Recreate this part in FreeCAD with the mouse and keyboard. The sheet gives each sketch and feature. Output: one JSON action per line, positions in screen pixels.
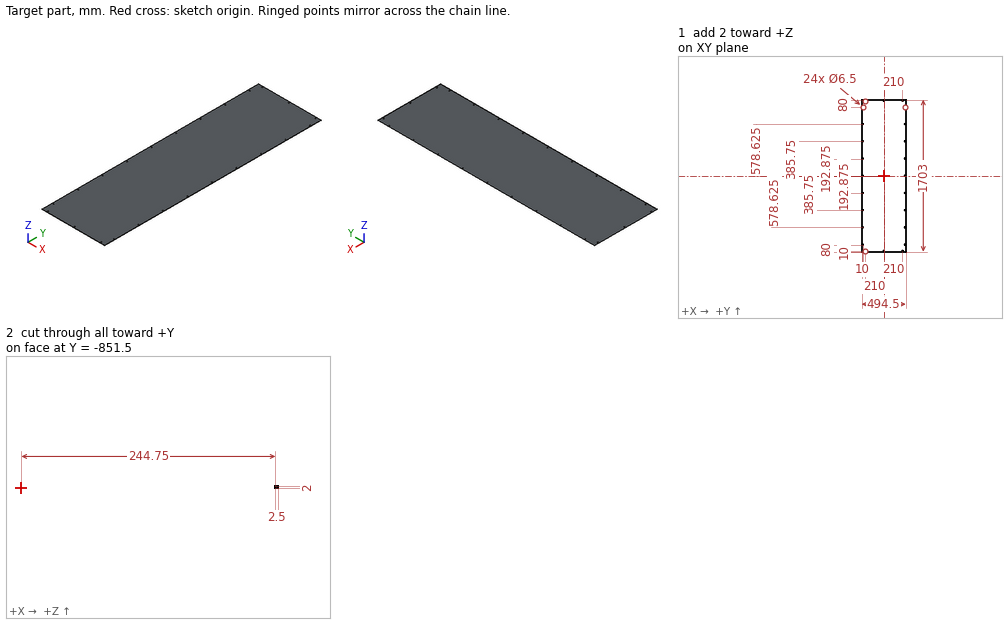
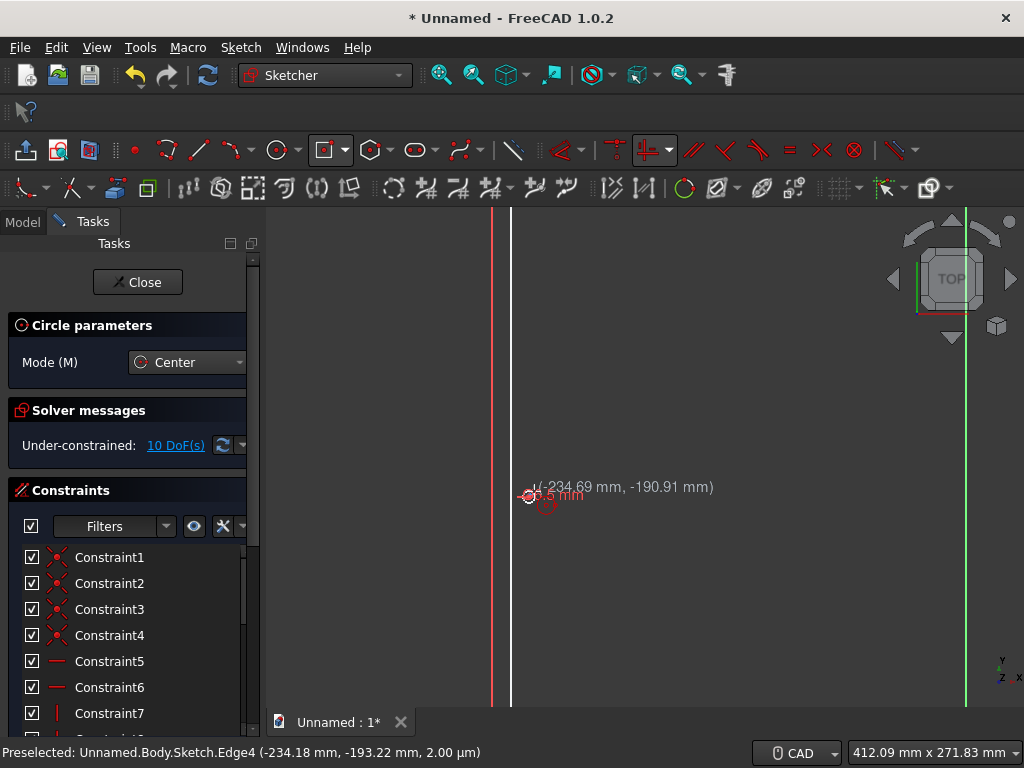
{"action": "scroll", "coordinate": [538, 489], "scroll_direction": "down", "scroll_amount": 12}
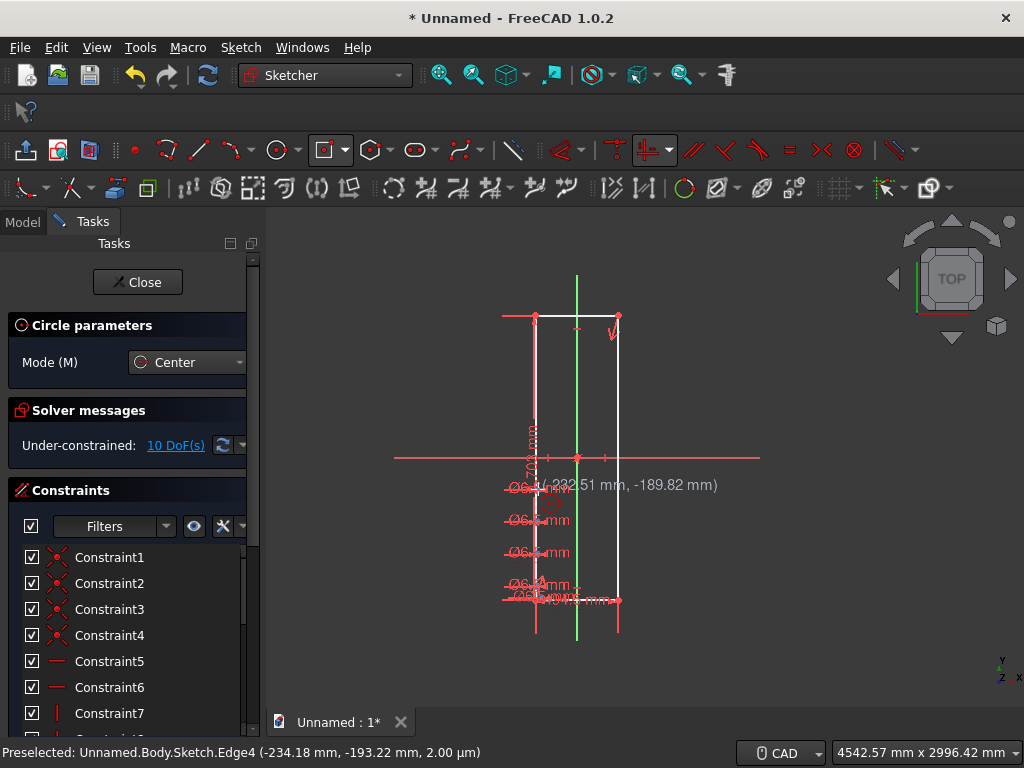
{"action": "scroll", "coordinate": [577, 598], "scroll_direction": "up", "scroll_amount": 19}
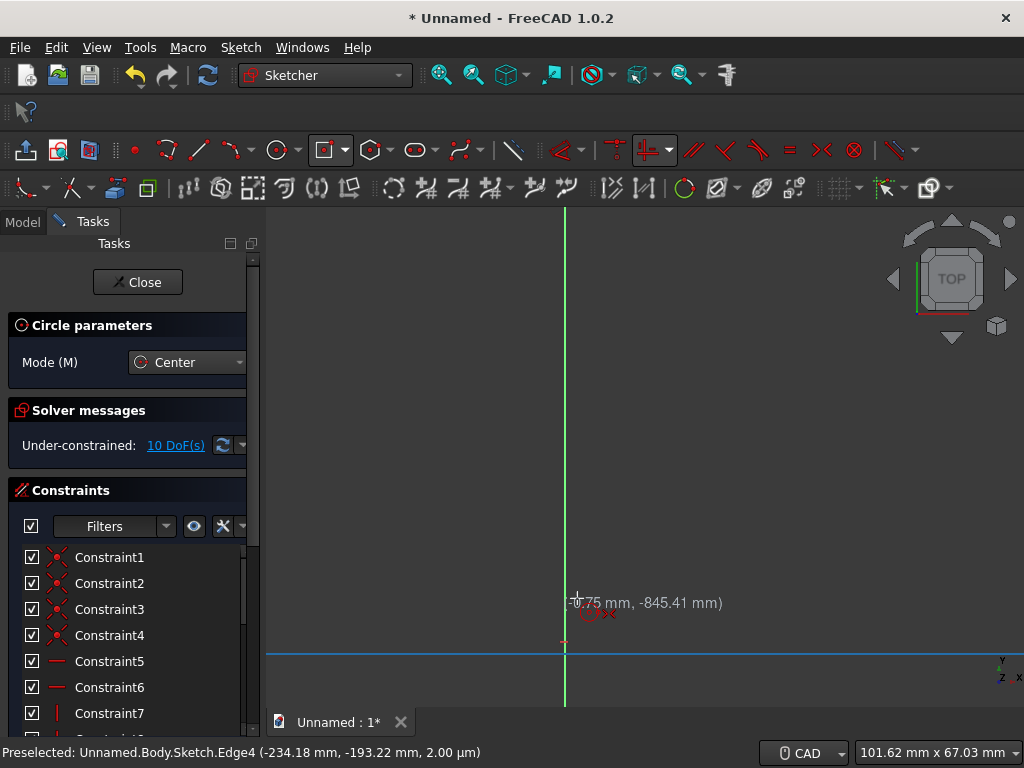
{"action": "scroll", "coordinate": [577, 630], "scroll_direction": "down", "scroll_amount": 18}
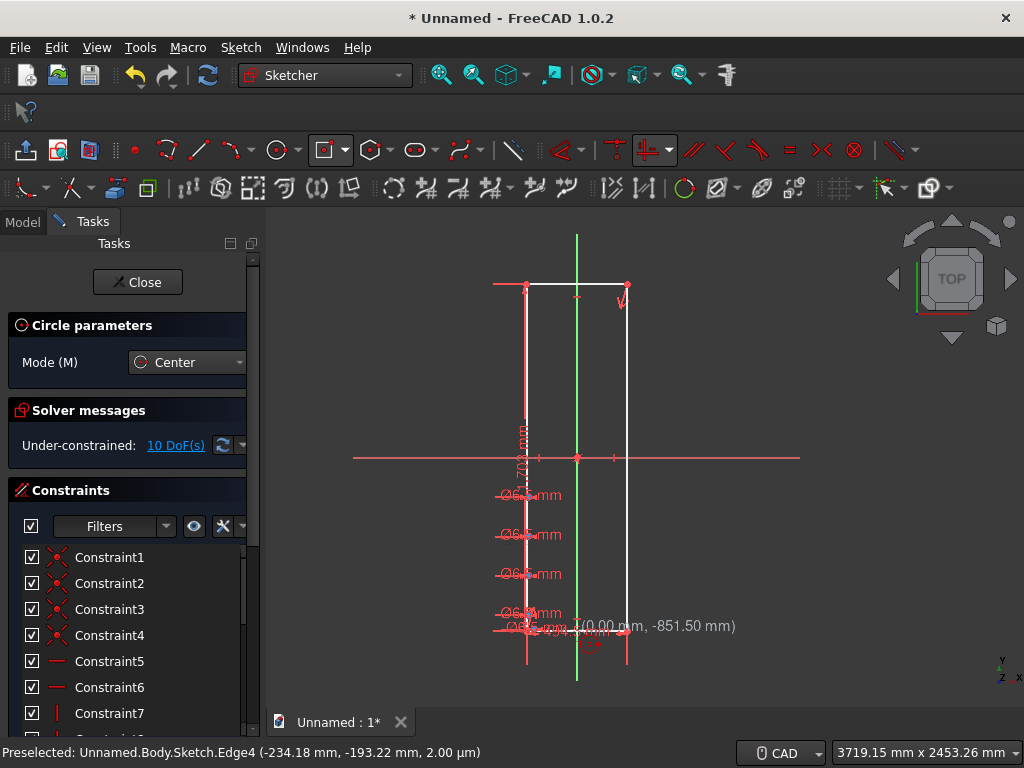
{"action": "scroll", "coordinate": [577, 629], "scroll_direction": "up", "scroll_amount": 11}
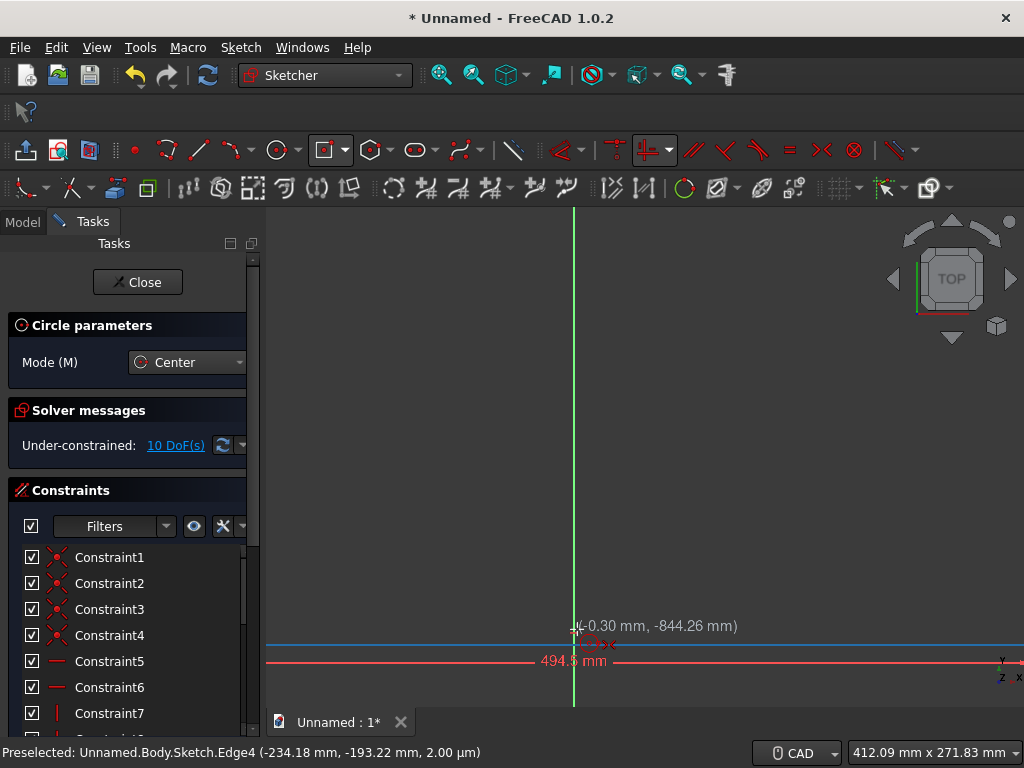
{"action": "left_click", "coordinate": [574, 626]}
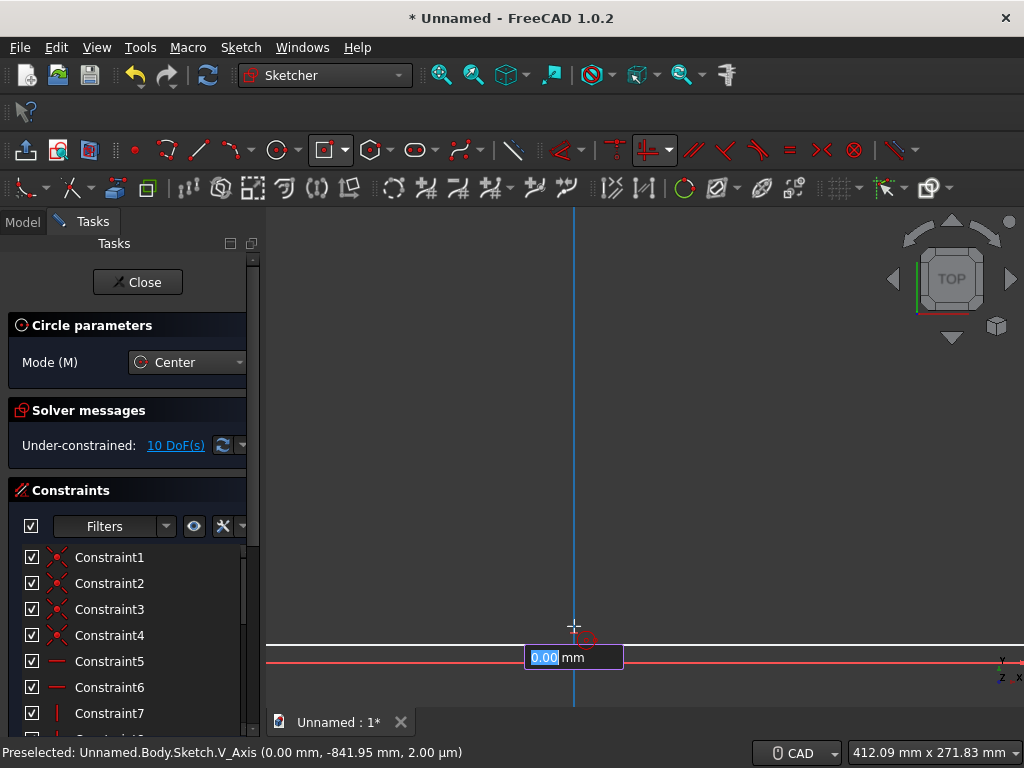
{"action": "scroll", "coordinate": [580, 624], "scroll_direction": "up", "scroll_amount": 6}
{"action": "mouse_move", "coordinate": [579, 622]}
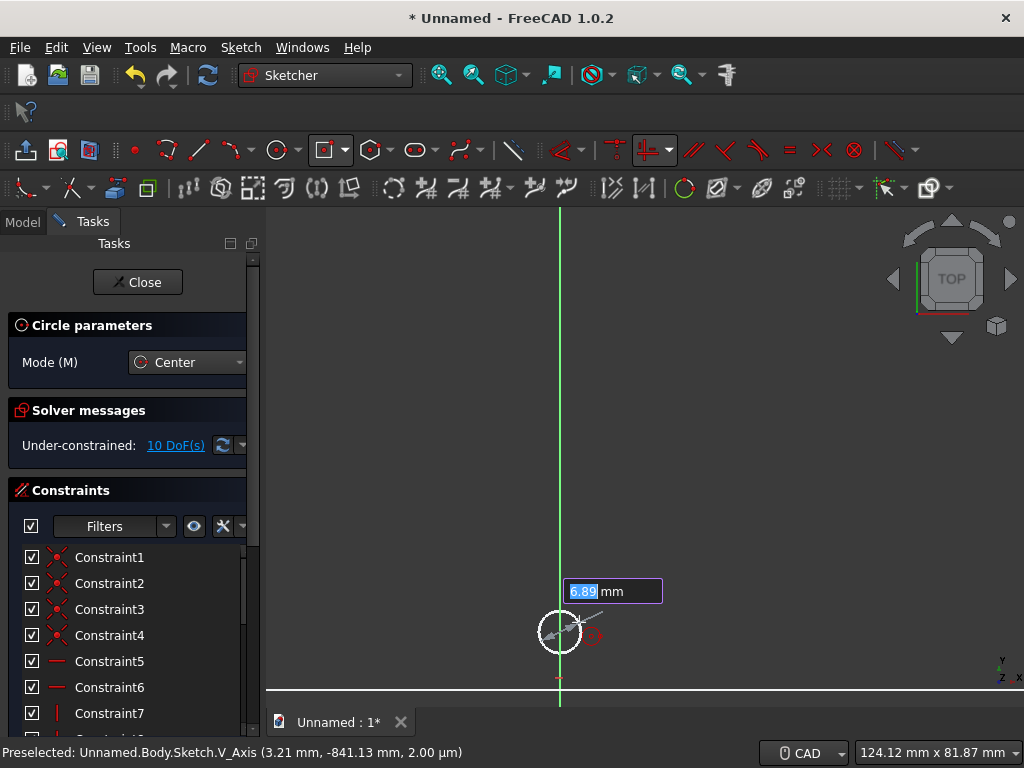
{"action": "type", "text": "6.5"}
{"action": "key", "text": "Return"}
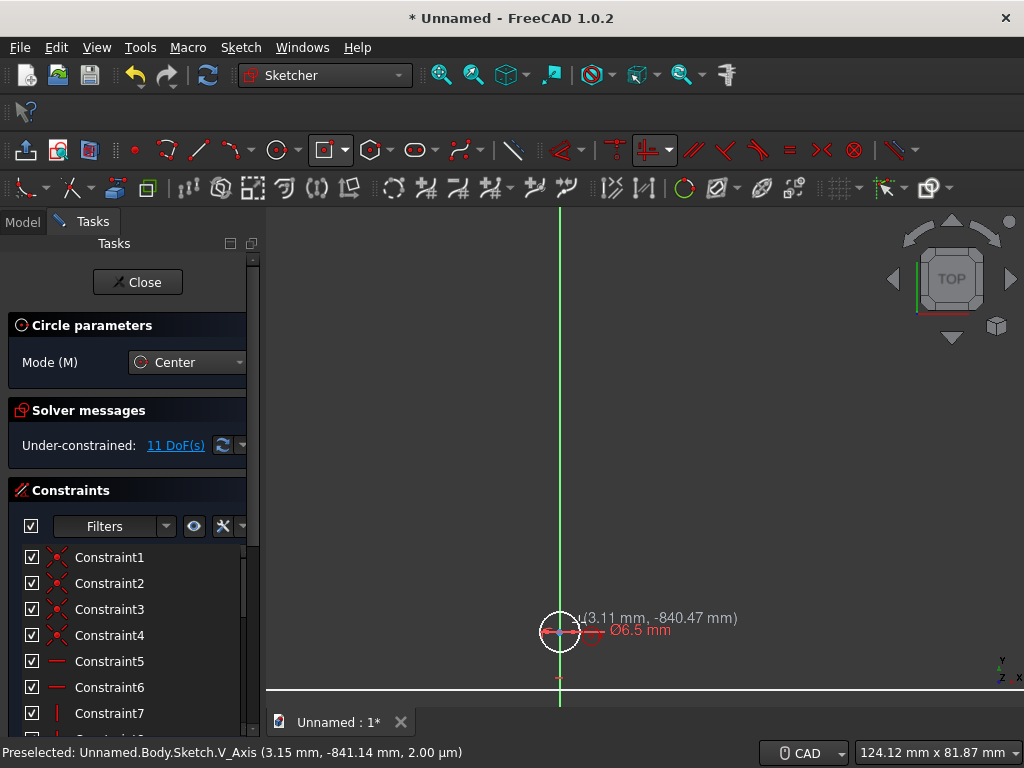
{"action": "scroll", "coordinate": [577, 628], "scroll_direction": "down", "scroll_amount": 17}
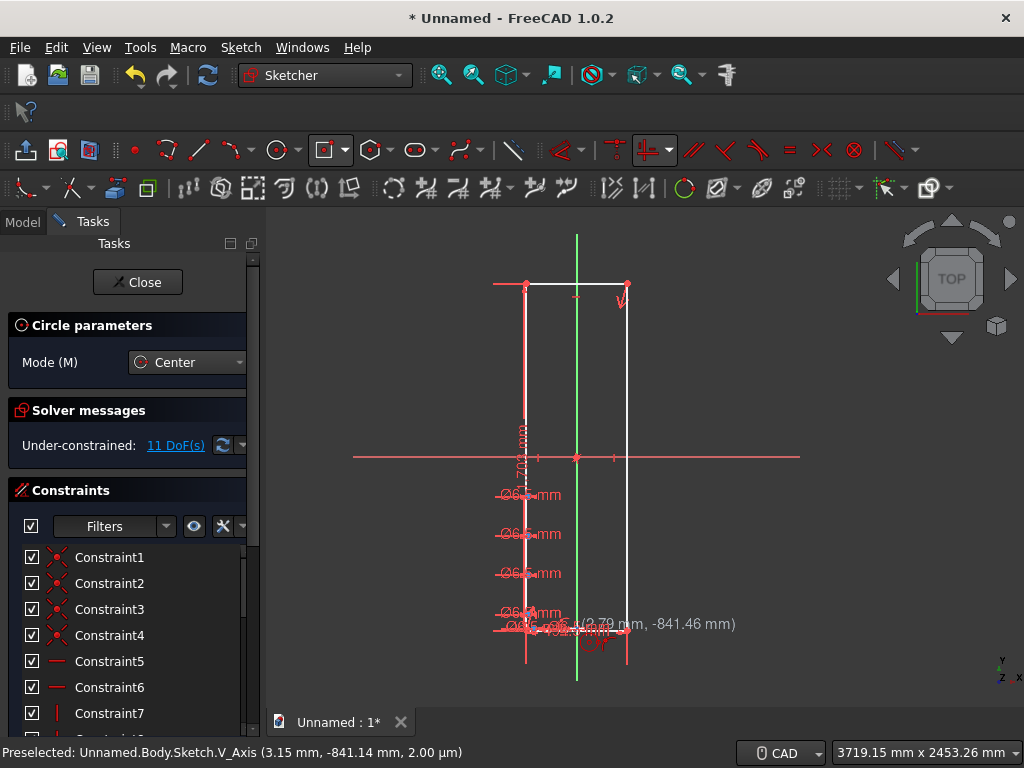
{"action": "scroll", "coordinate": [620, 629], "scroll_direction": "up", "scroll_amount": 18}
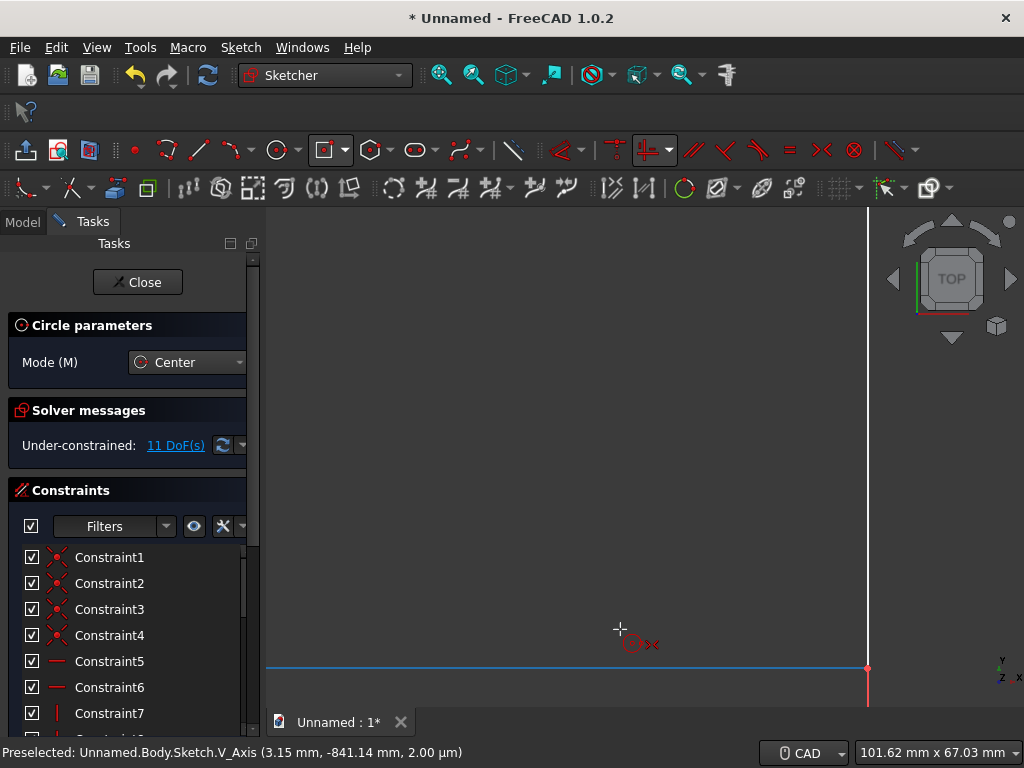
{"action": "scroll", "coordinate": [620, 629], "scroll_direction": "down", "scroll_amount": 18}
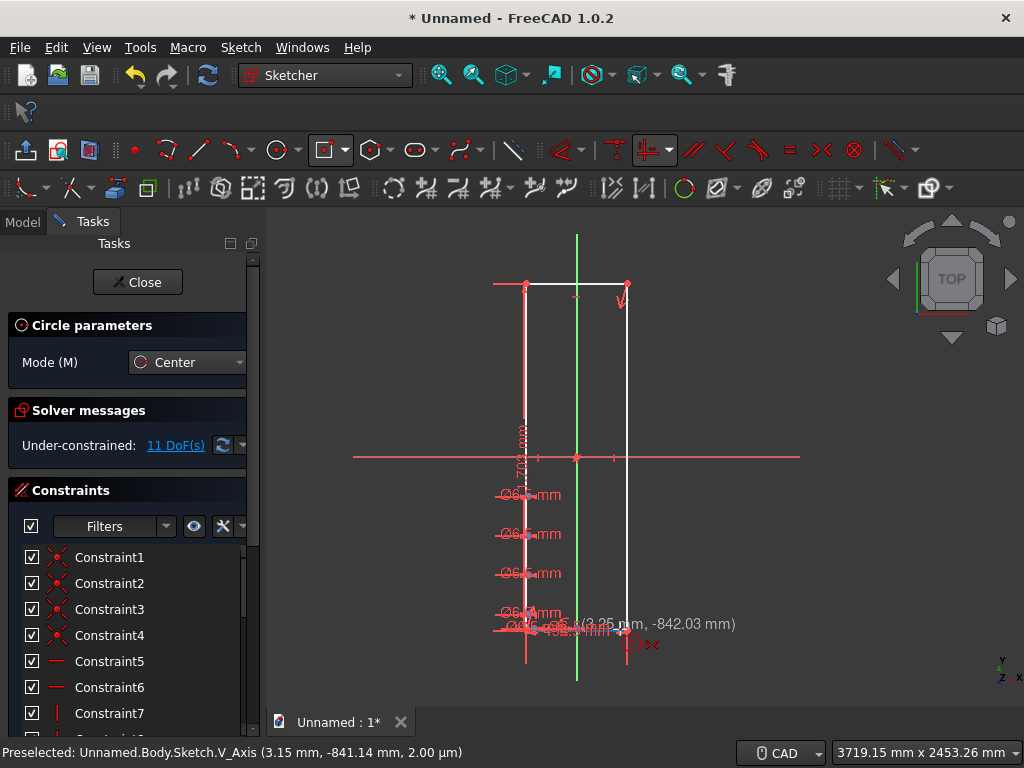
{"action": "scroll", "coordinate": [620, 629], "scroll_direction": "up", "scroll_amount": 11}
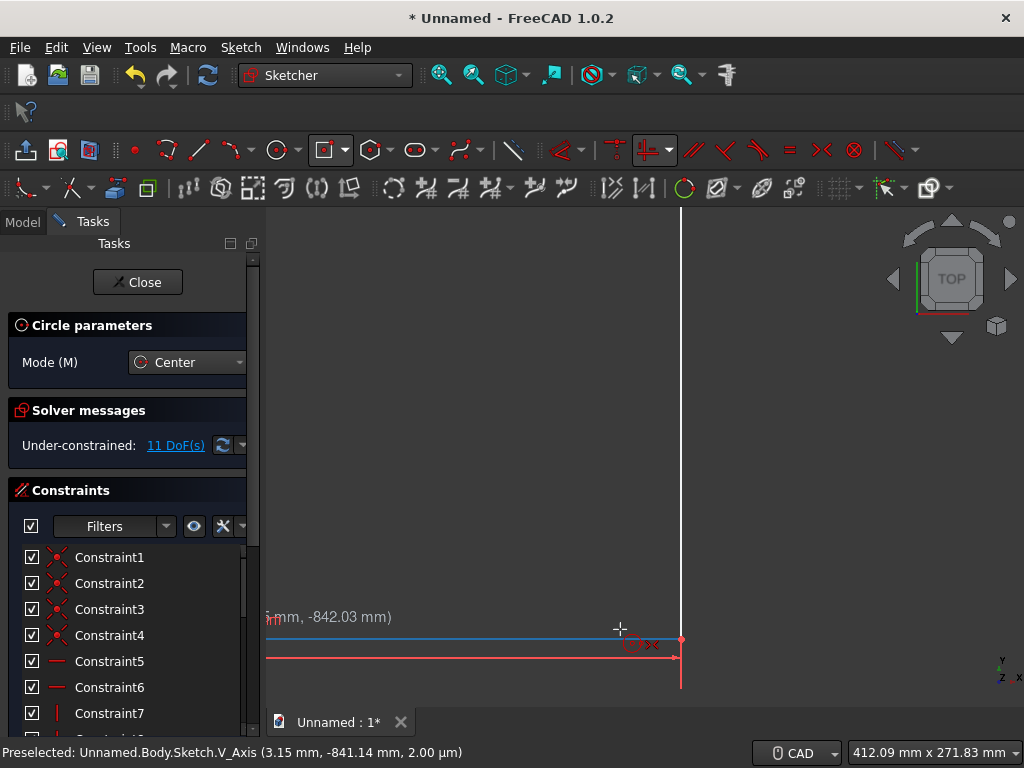
{"action": "left_click", "coordinate": [613, 621]}
{"action": "mouse_move", "coordinate": [617, 617]}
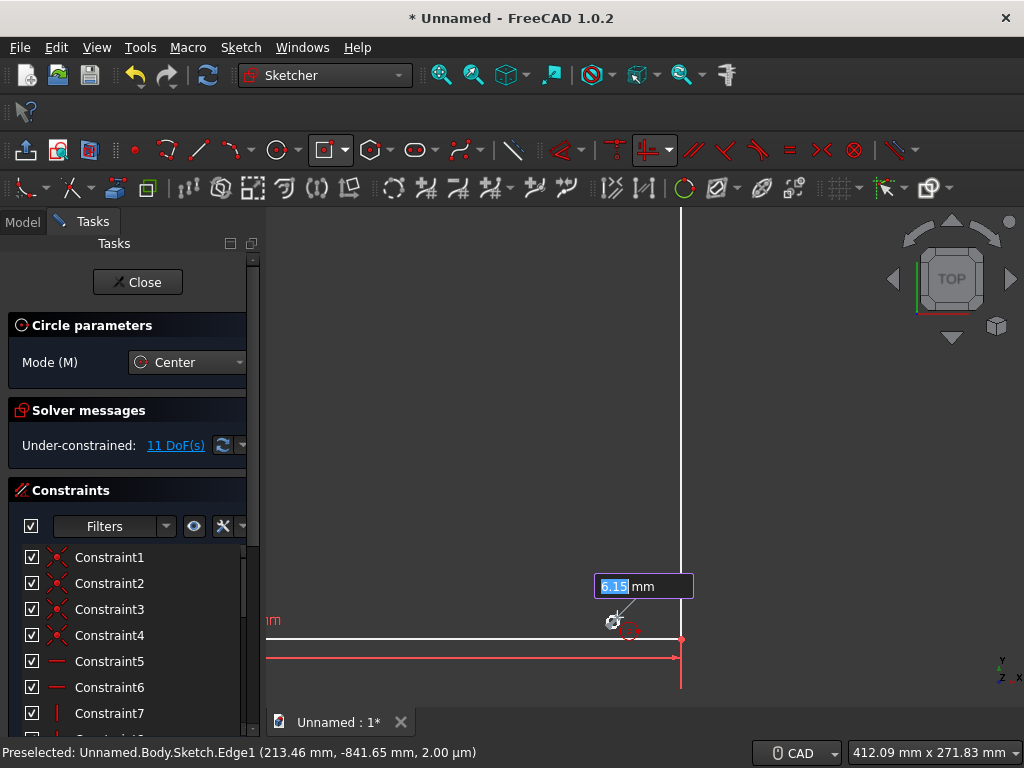
{"action": "type", "text": "6.5"}
{"action": "key", "text": "Return"}